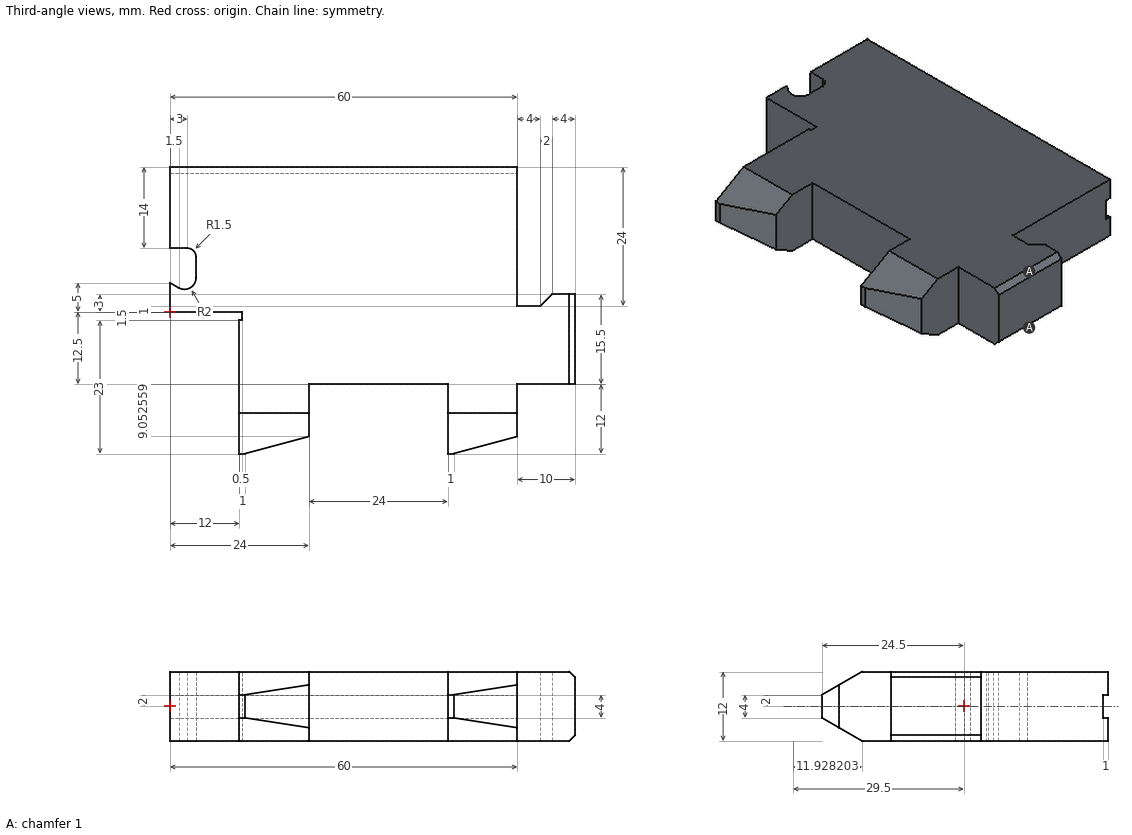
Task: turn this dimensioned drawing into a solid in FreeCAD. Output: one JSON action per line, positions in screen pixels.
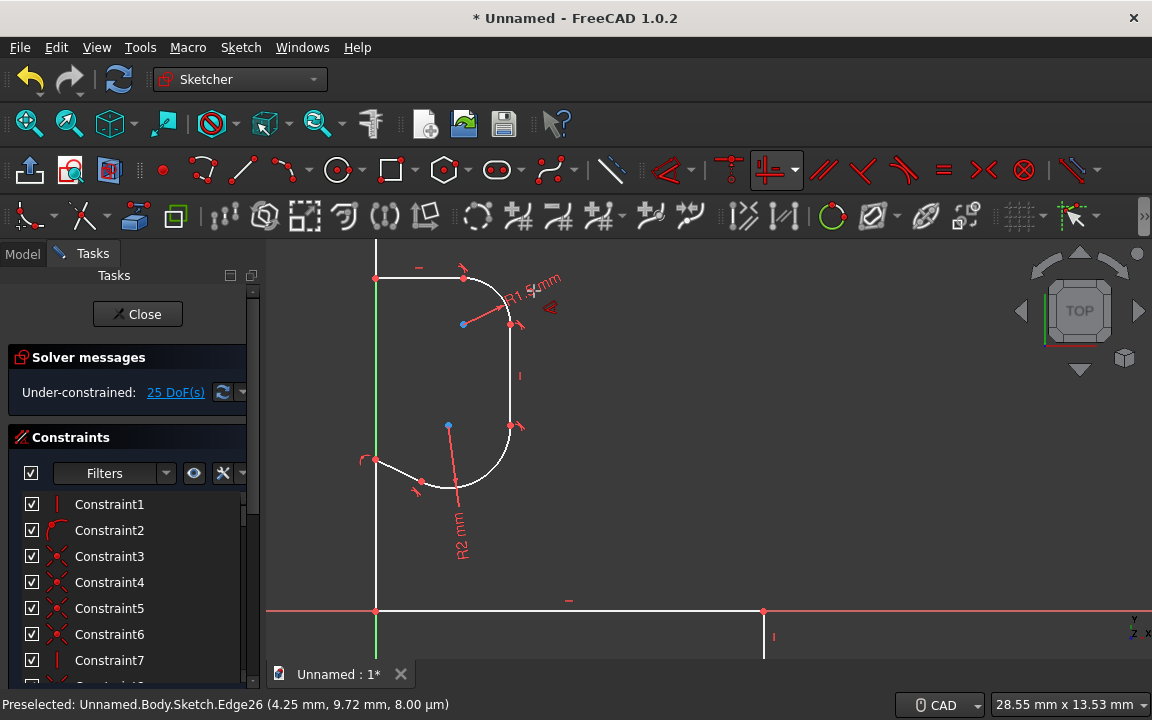
{"action": "scroll", "coordinate": [478, 418], "scroll_direction": "down", "scroll_amount": 9}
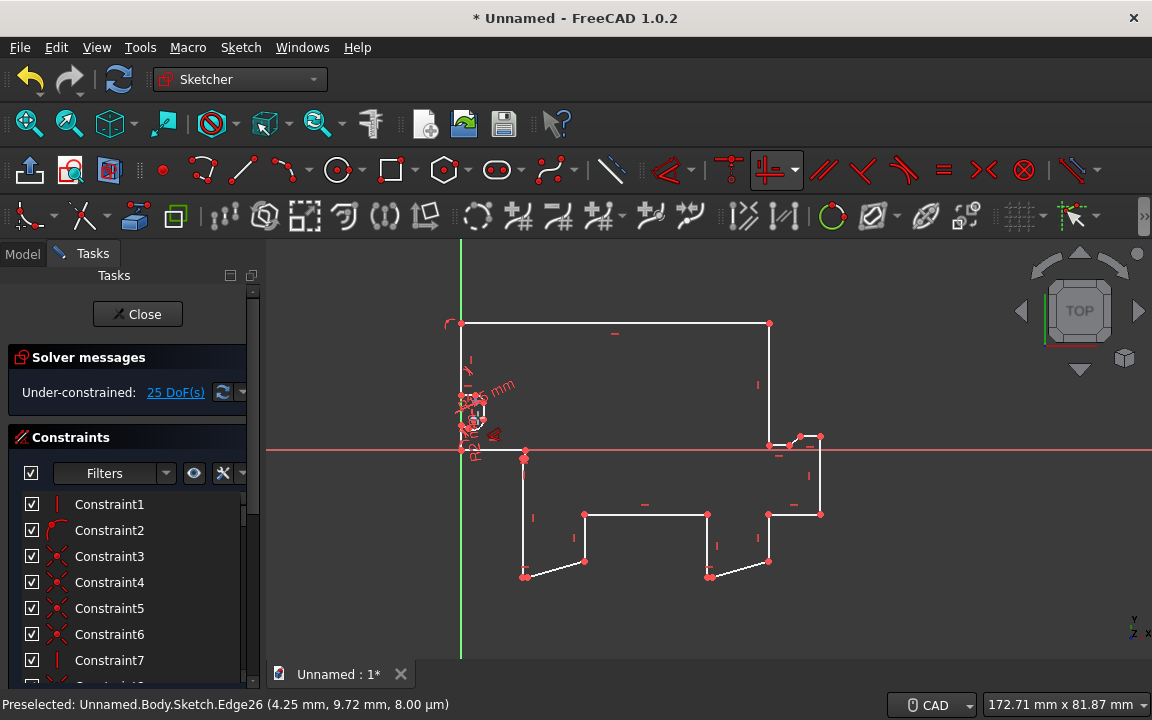
{"action": "scroll", "coordinate": [461, 433], "scroll_direction": "up", "scroll_amount": 4}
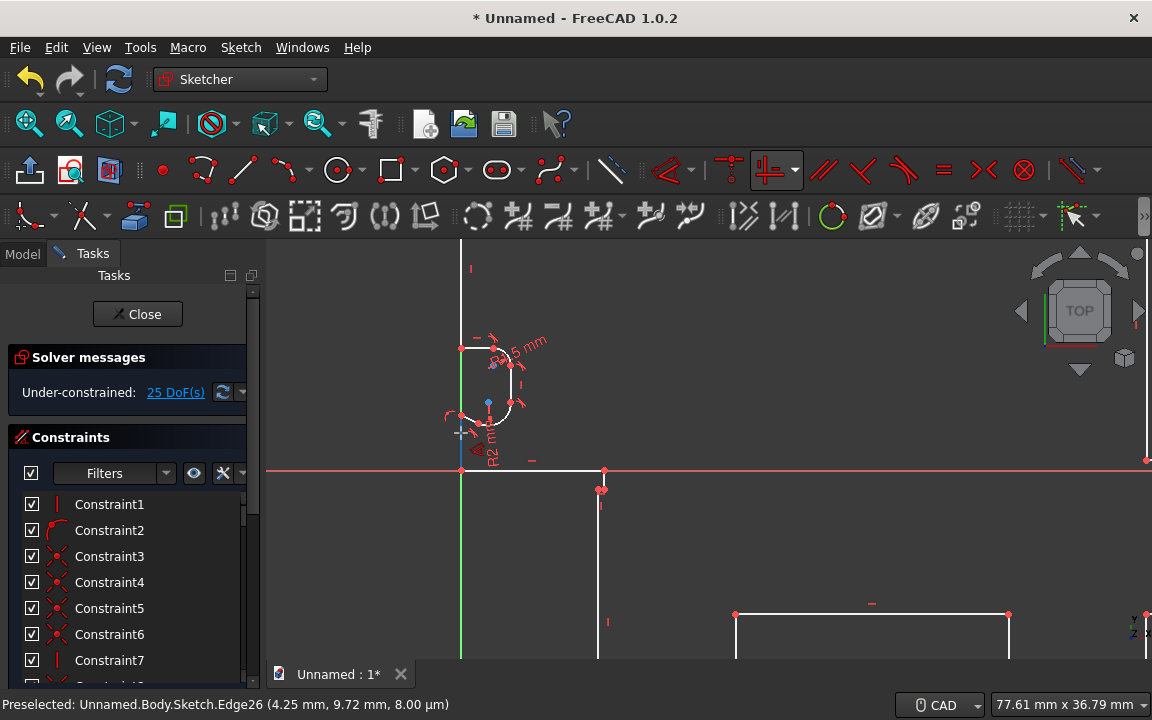
{"action": "left_click", "coordinate": [461, 432]}
{"action": "left_click", "coordinate": [427, 424]}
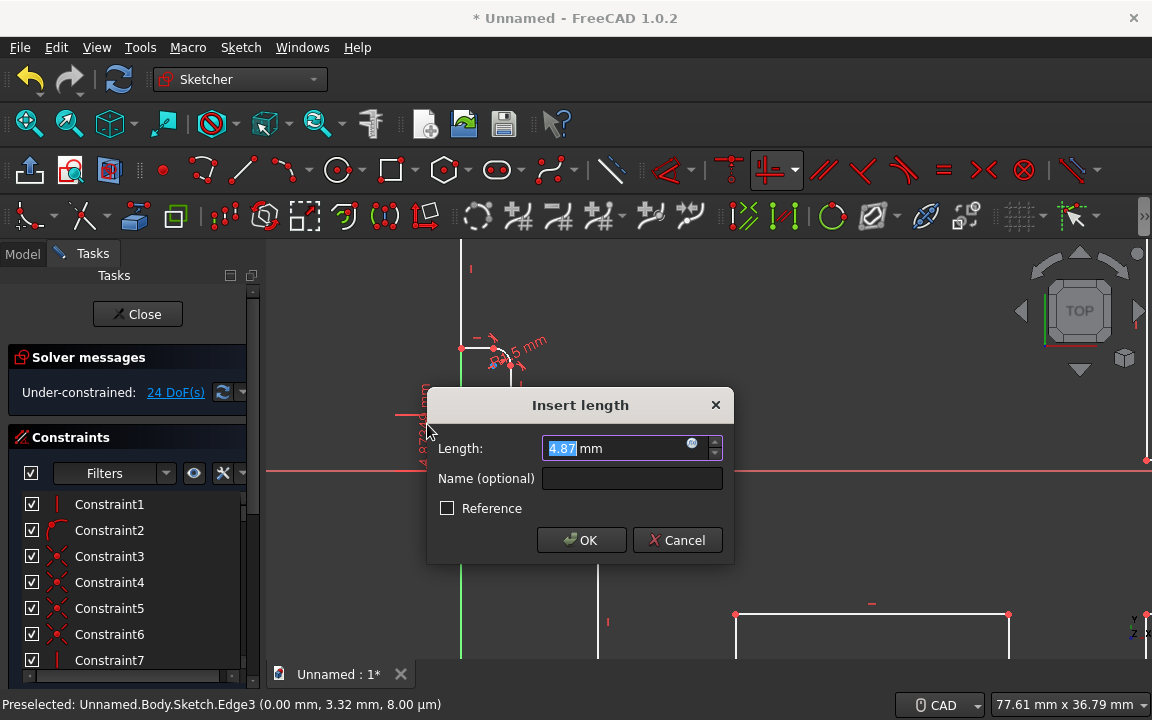
{"action": "type", "text": "5"}
{"action": "key", "text": "Return"}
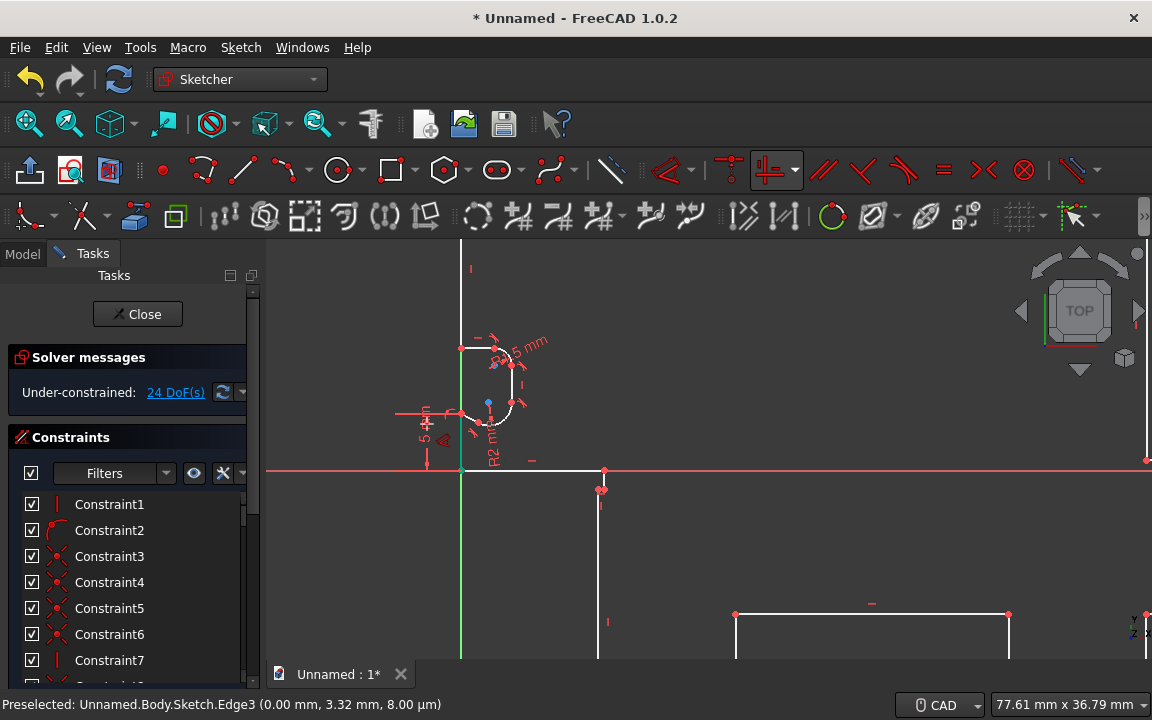
{"action": "scroll", "coordinate": [461, 433], "scroll_direction": "down", "scroll_amount": 4}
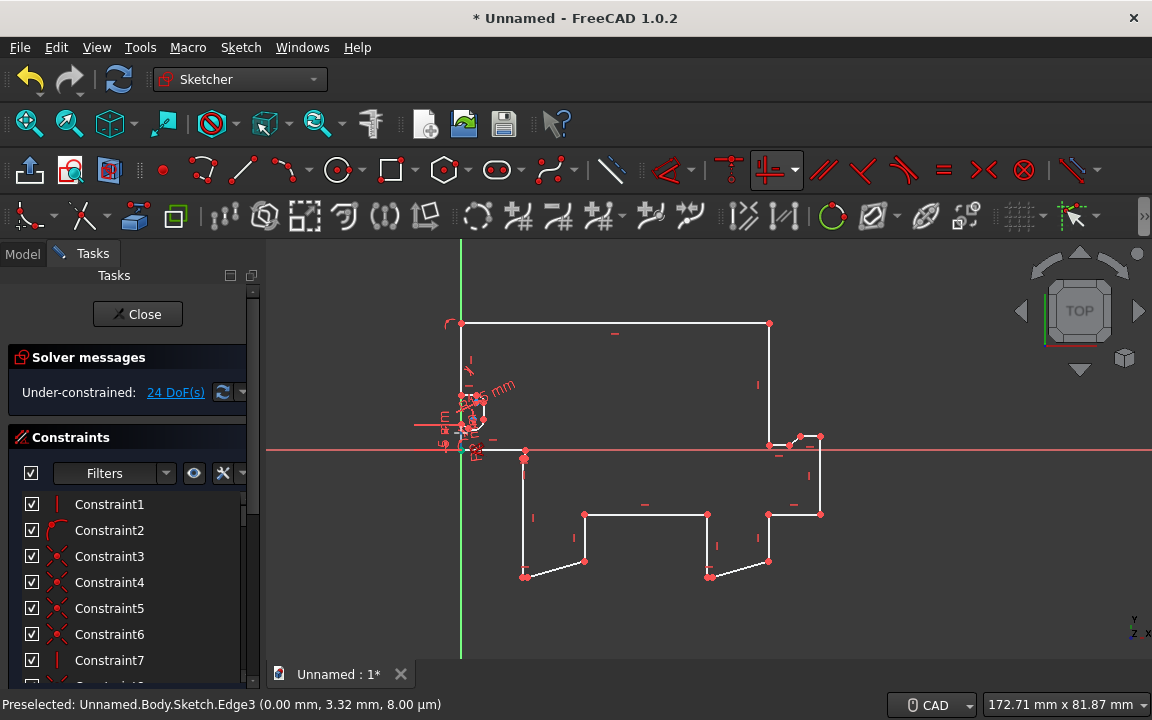
{"action": "scroll", "coordinate": [525, 577], "scroll_direction": "up", "scroll_amount": 11}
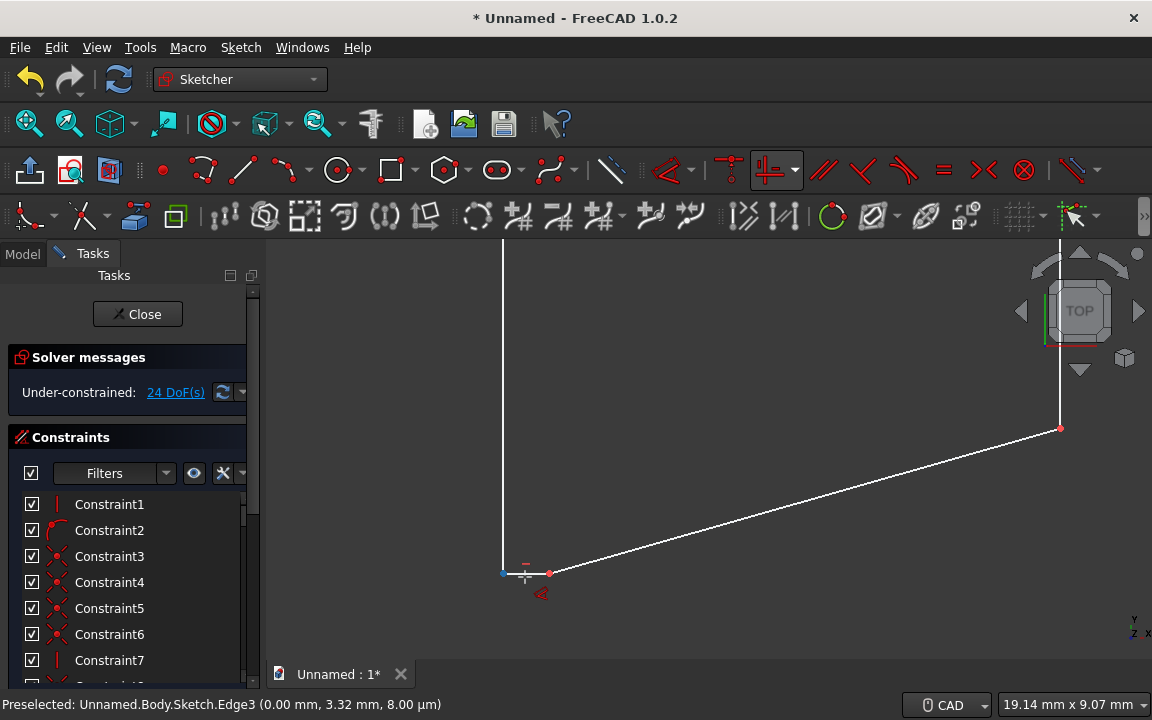
{"action": "left_click", "coordinate": [526, 574]}
{"action": "left_click", "coordinate": [526, 608]}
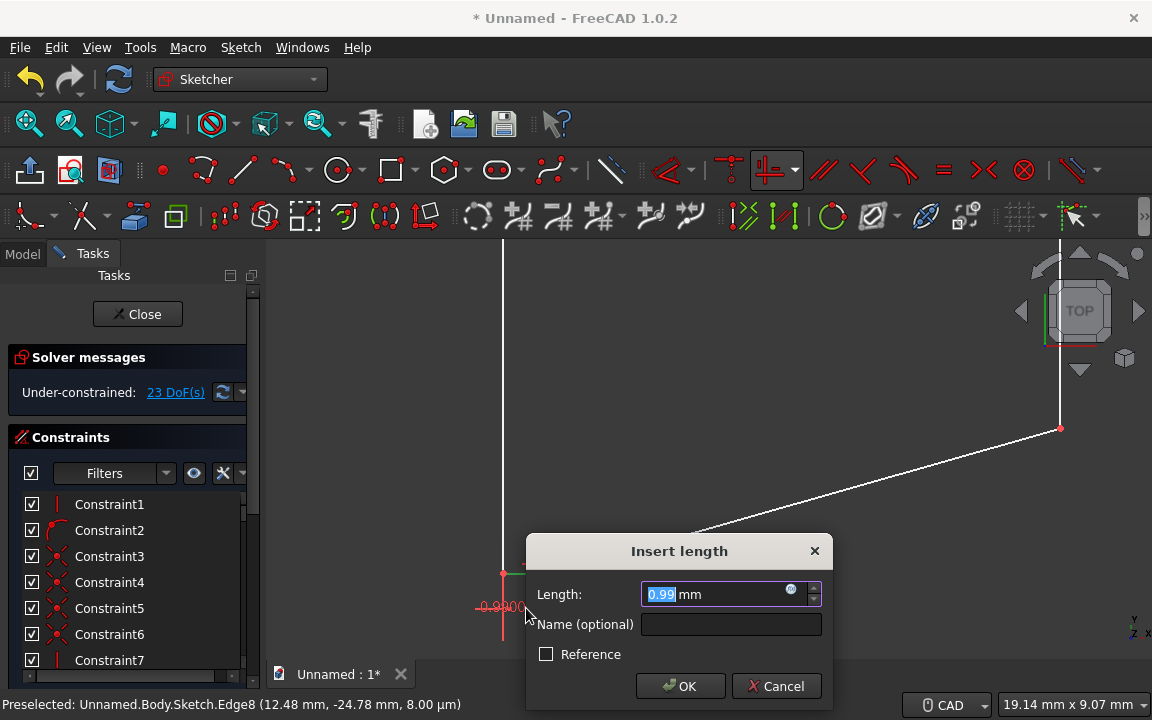
{"action": "type", "text": "1"}
{"action": "key", "text": "Return"}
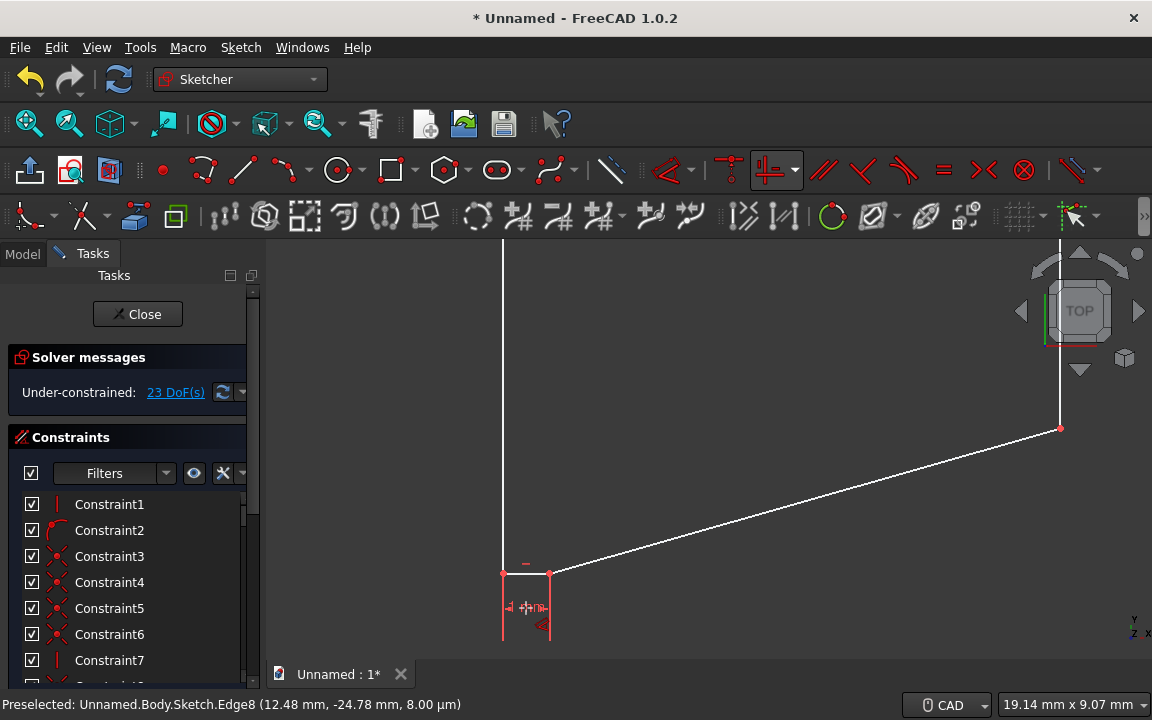
{"action": "scroll", "coordinate": [525, 578], "scroll_direction": "down", "scroll_amount": 11}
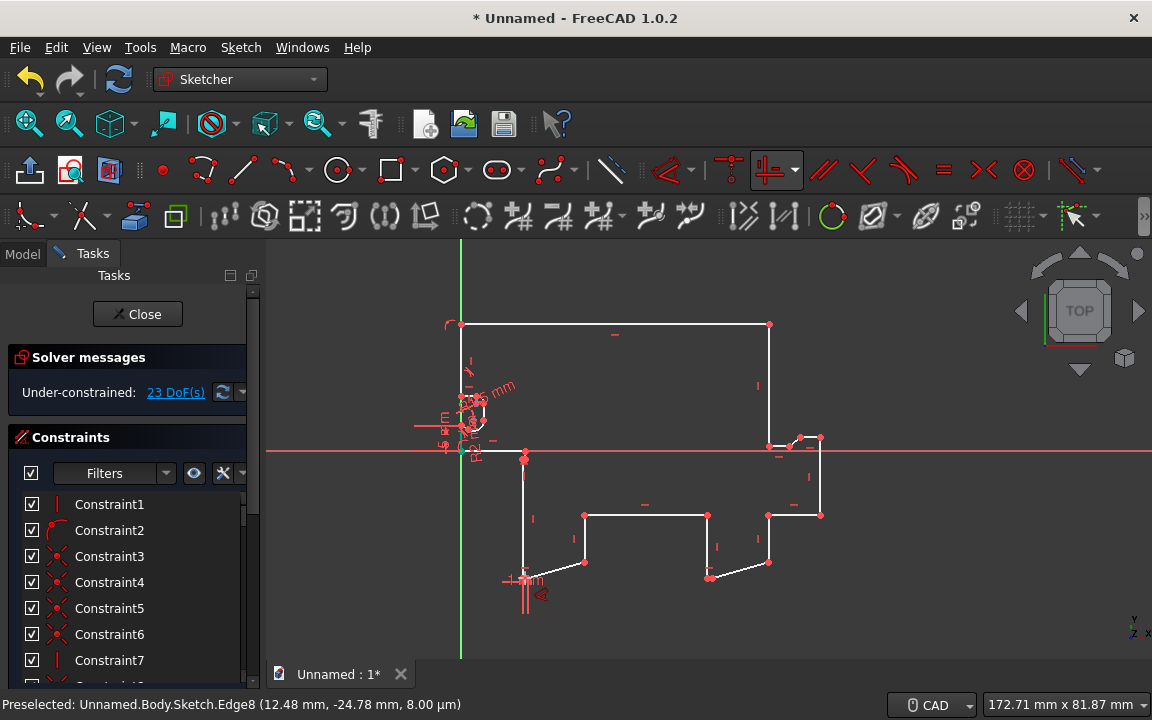
{"action": "scroll", "coordinate": [709, 578], "scroll_direction": "up", "scroll_amount": 11}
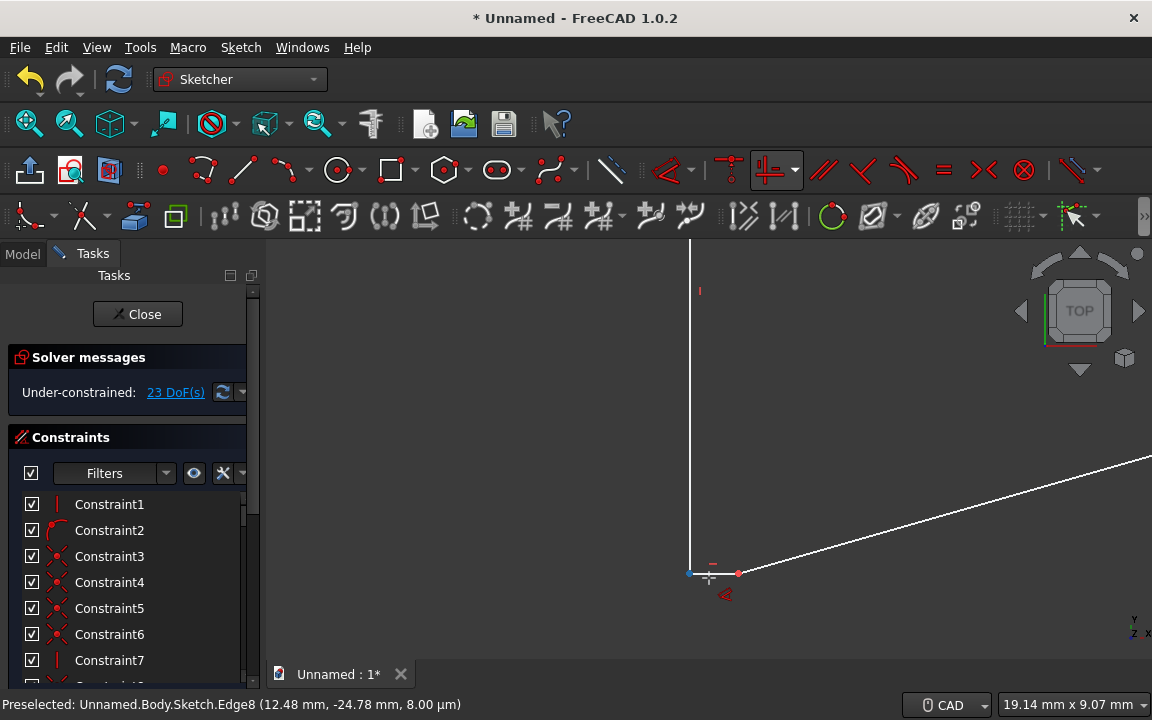
{"action": "left_click", "coordinate": [704, 574]}
{"action": "left_click", "coordinate": [714, 608]}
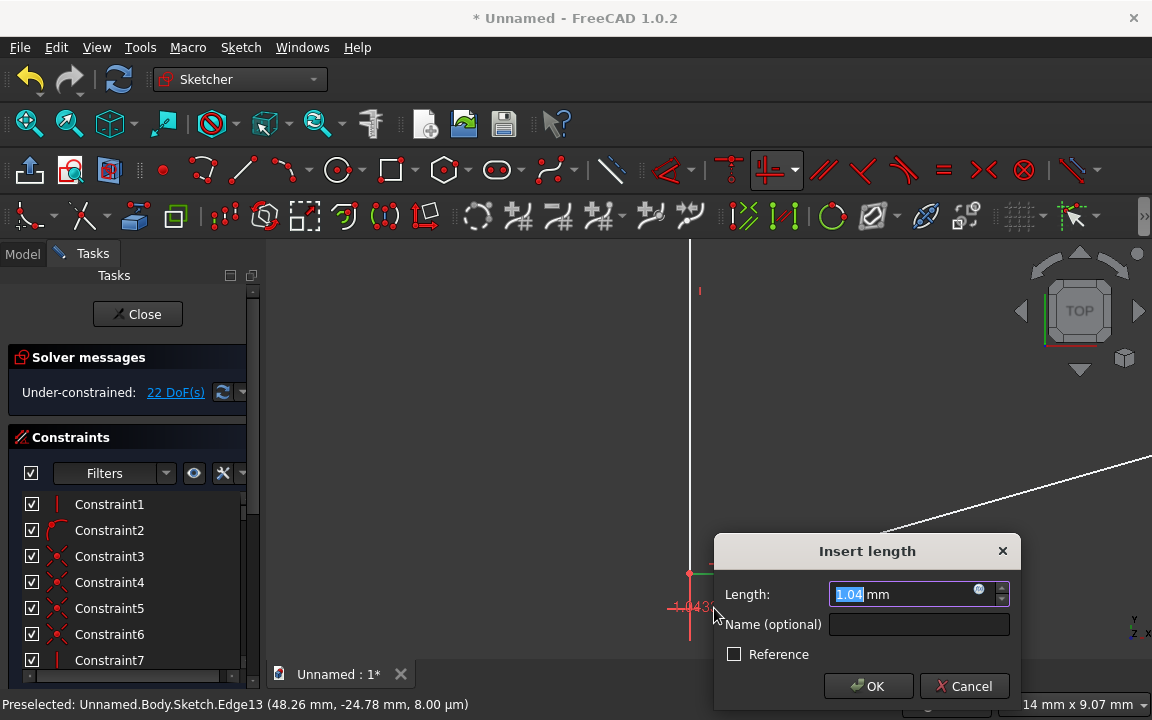
{"action": "type", "text": "1"}
{"action": "key", "text": "Return"}